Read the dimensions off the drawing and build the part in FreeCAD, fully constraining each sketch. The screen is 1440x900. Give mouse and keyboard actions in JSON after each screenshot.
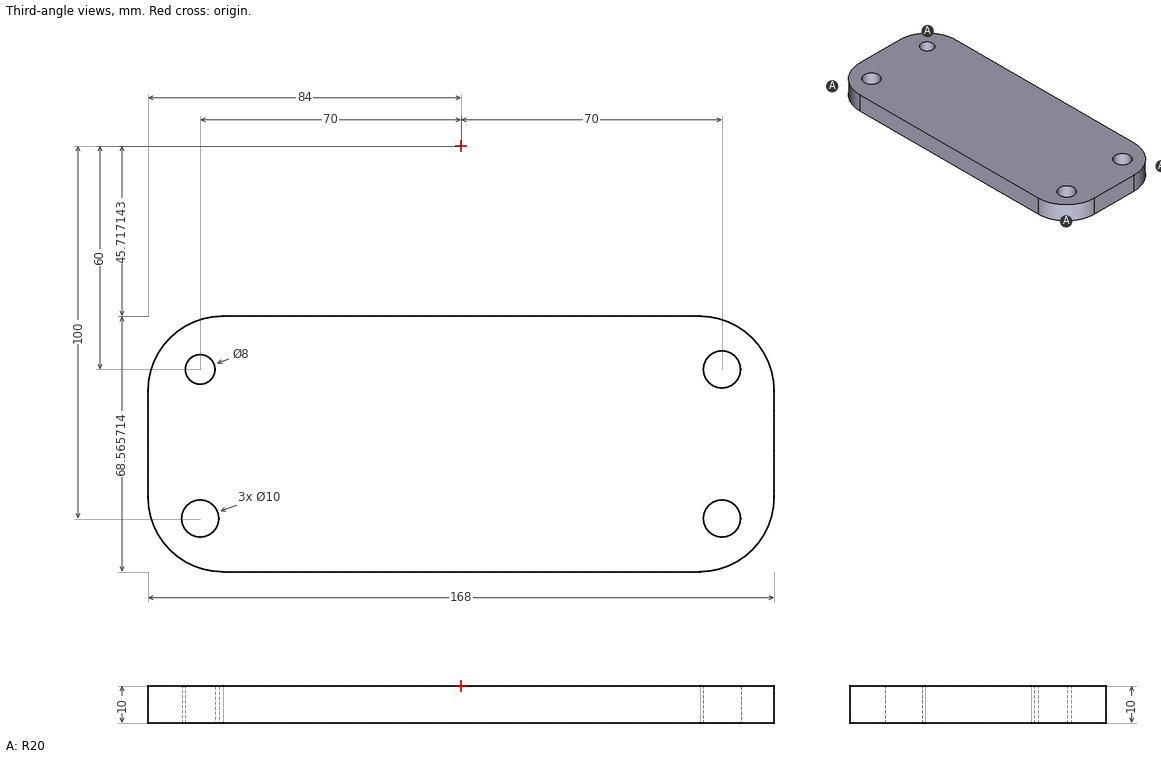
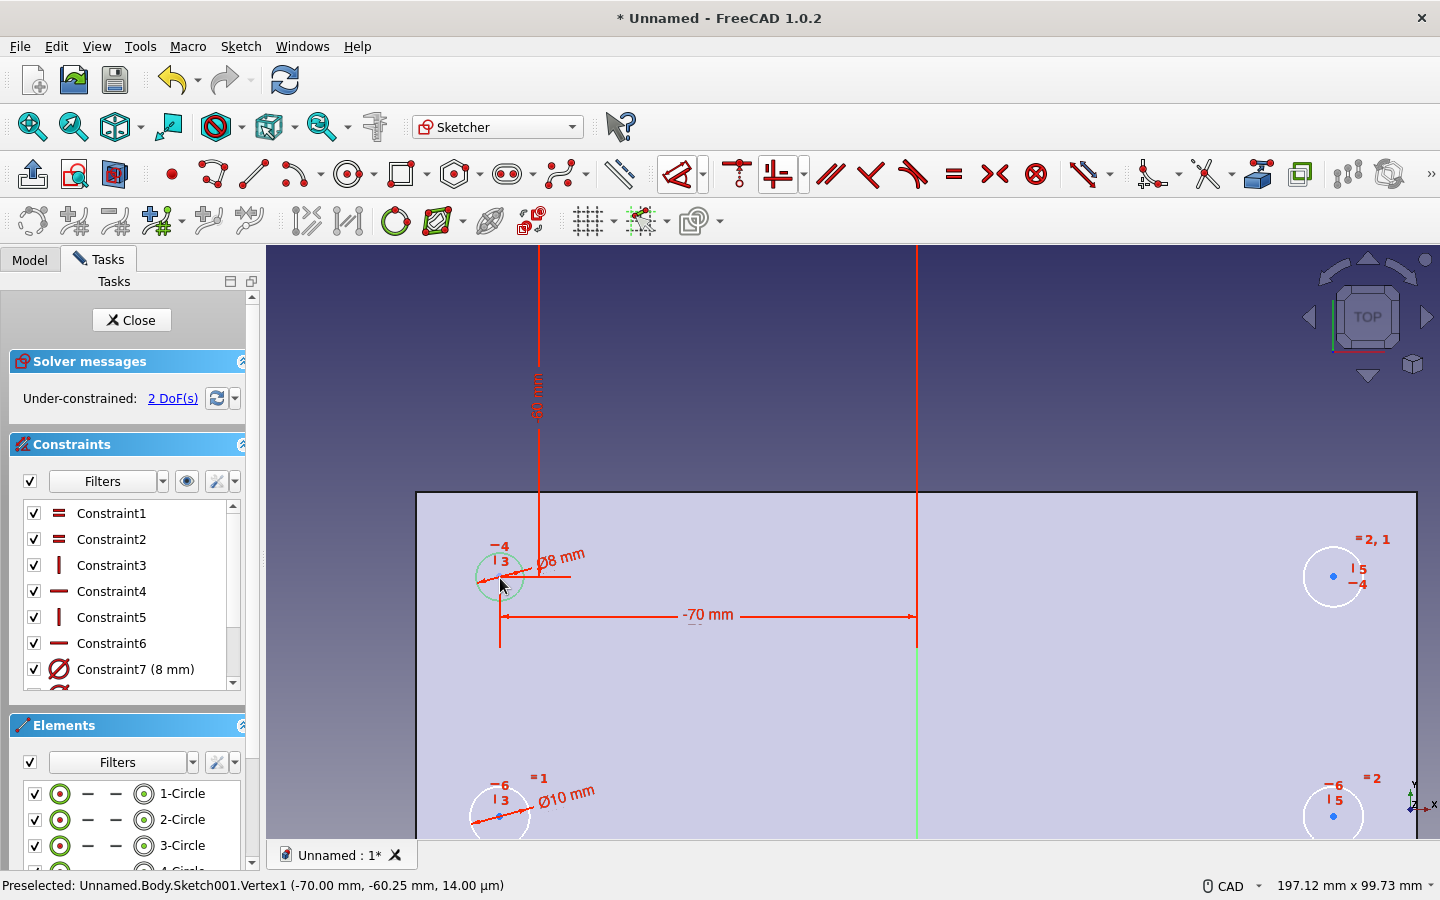
{"action": "scroll", "coordinate": [516, 562], "scroll_direction": "down", "scroll_amount": 2}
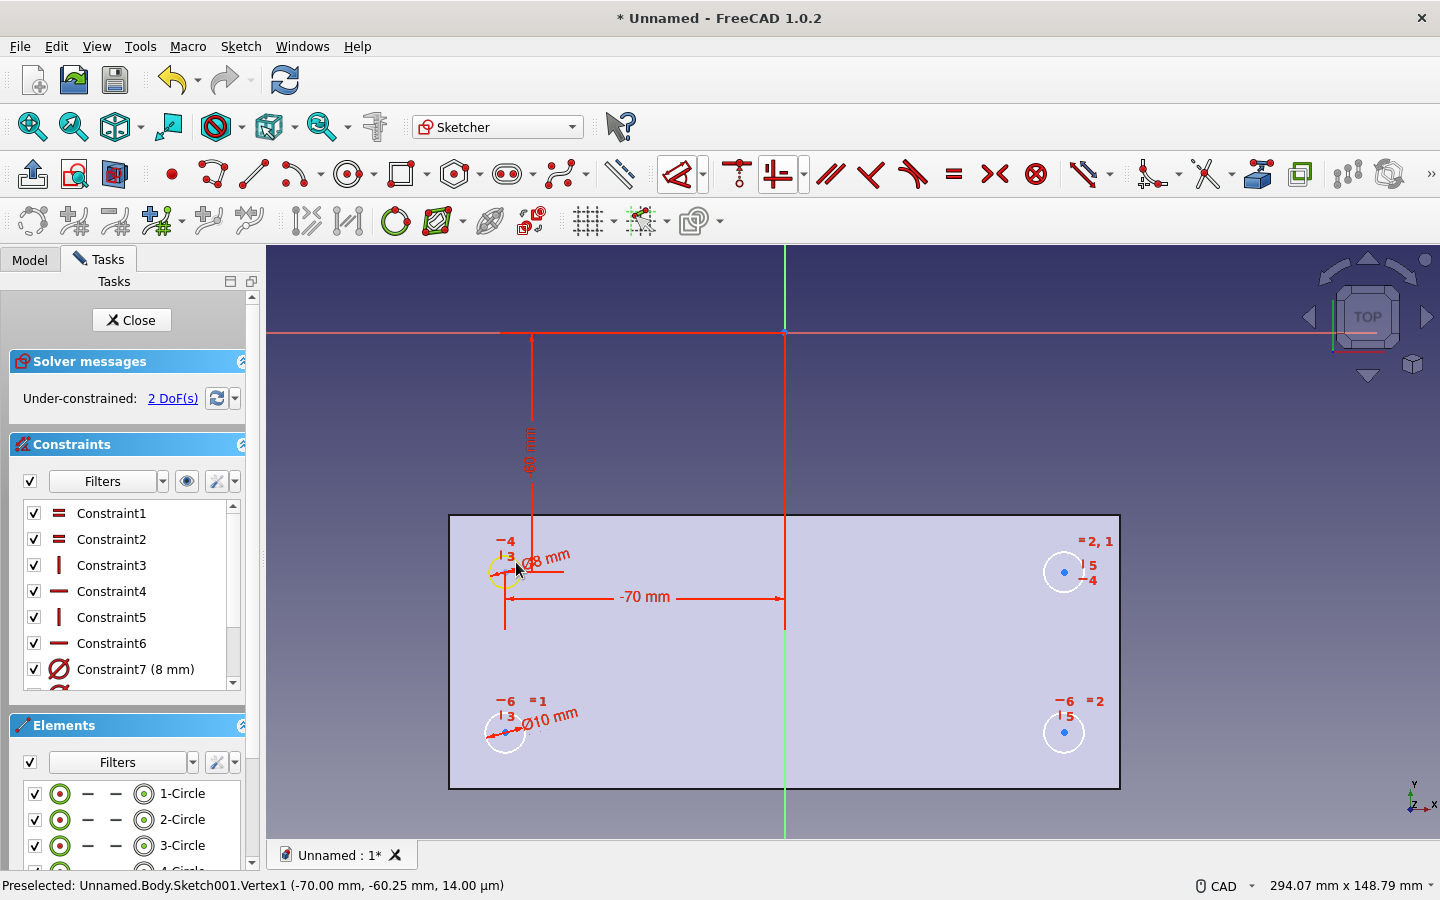
{"action": "left_click", "coordinate": [1064, 572]}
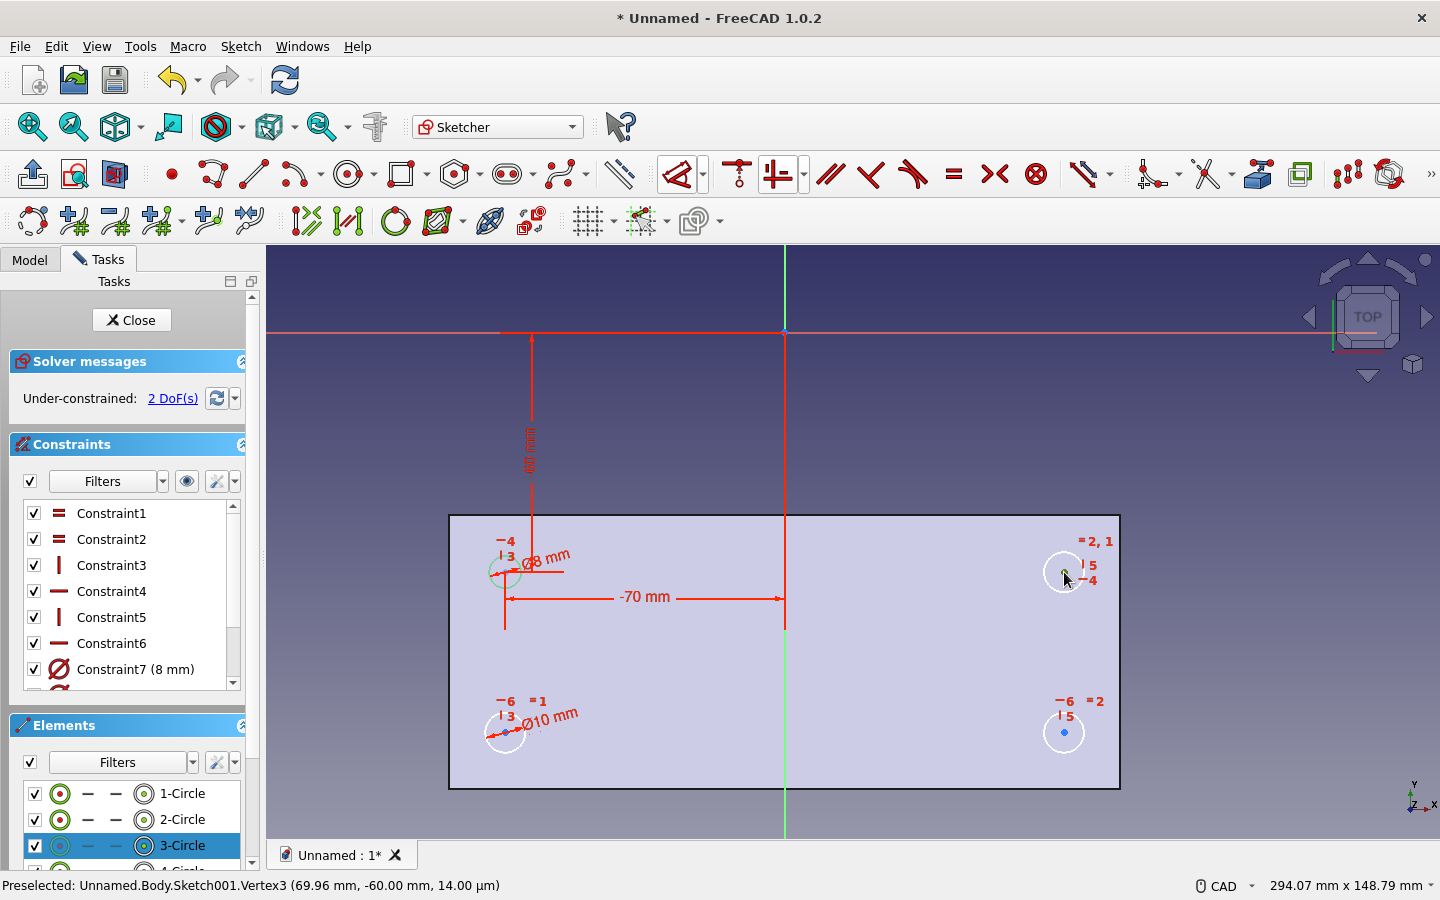
{"action": "left_click", "coordinate": [702, 174]}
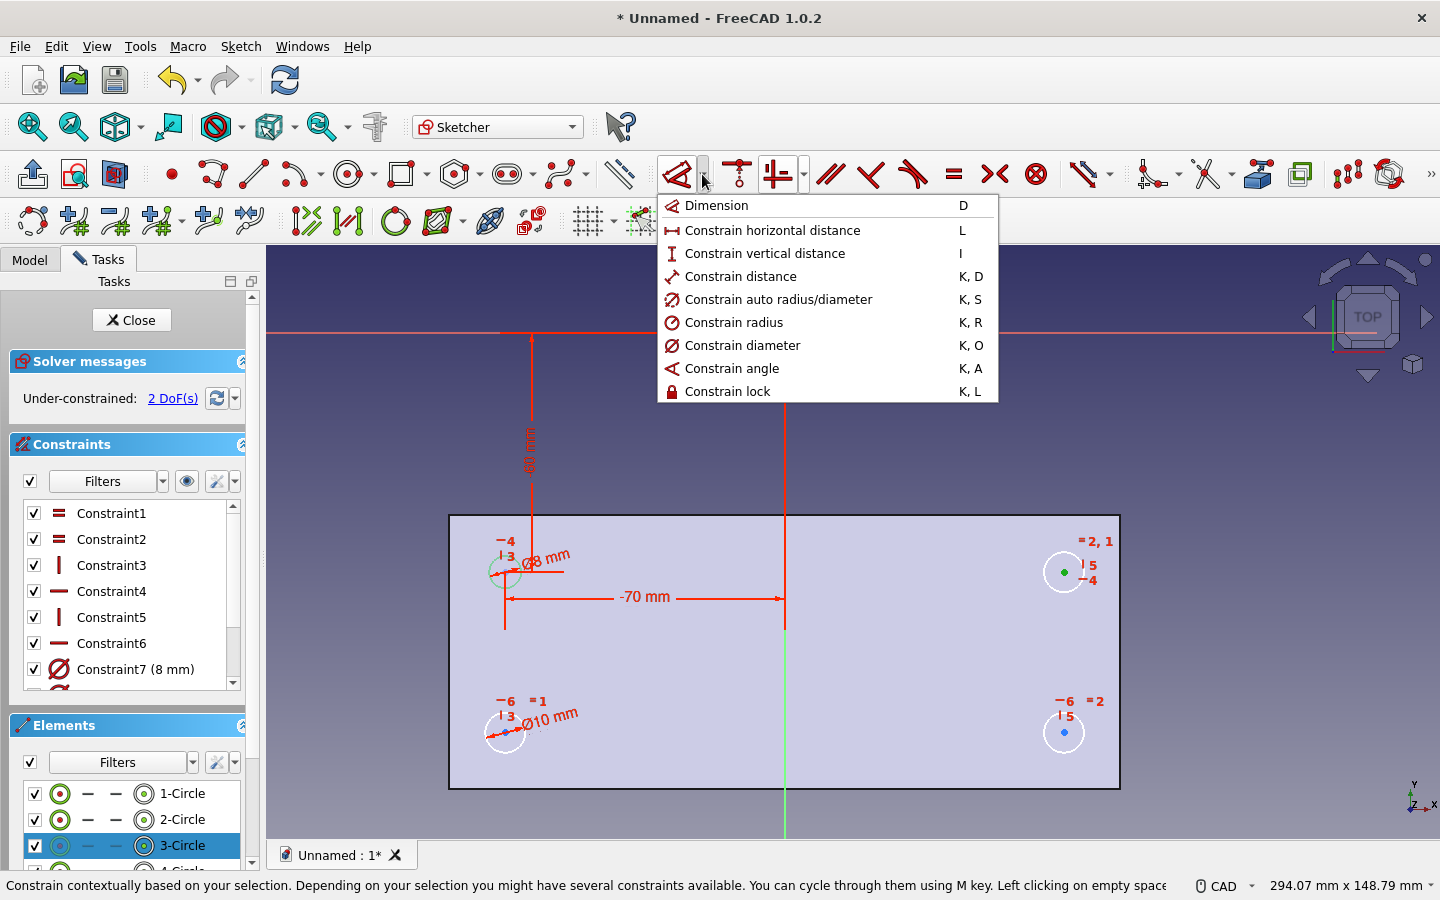
{"action": "left_click", "coordinate": [828, 230]}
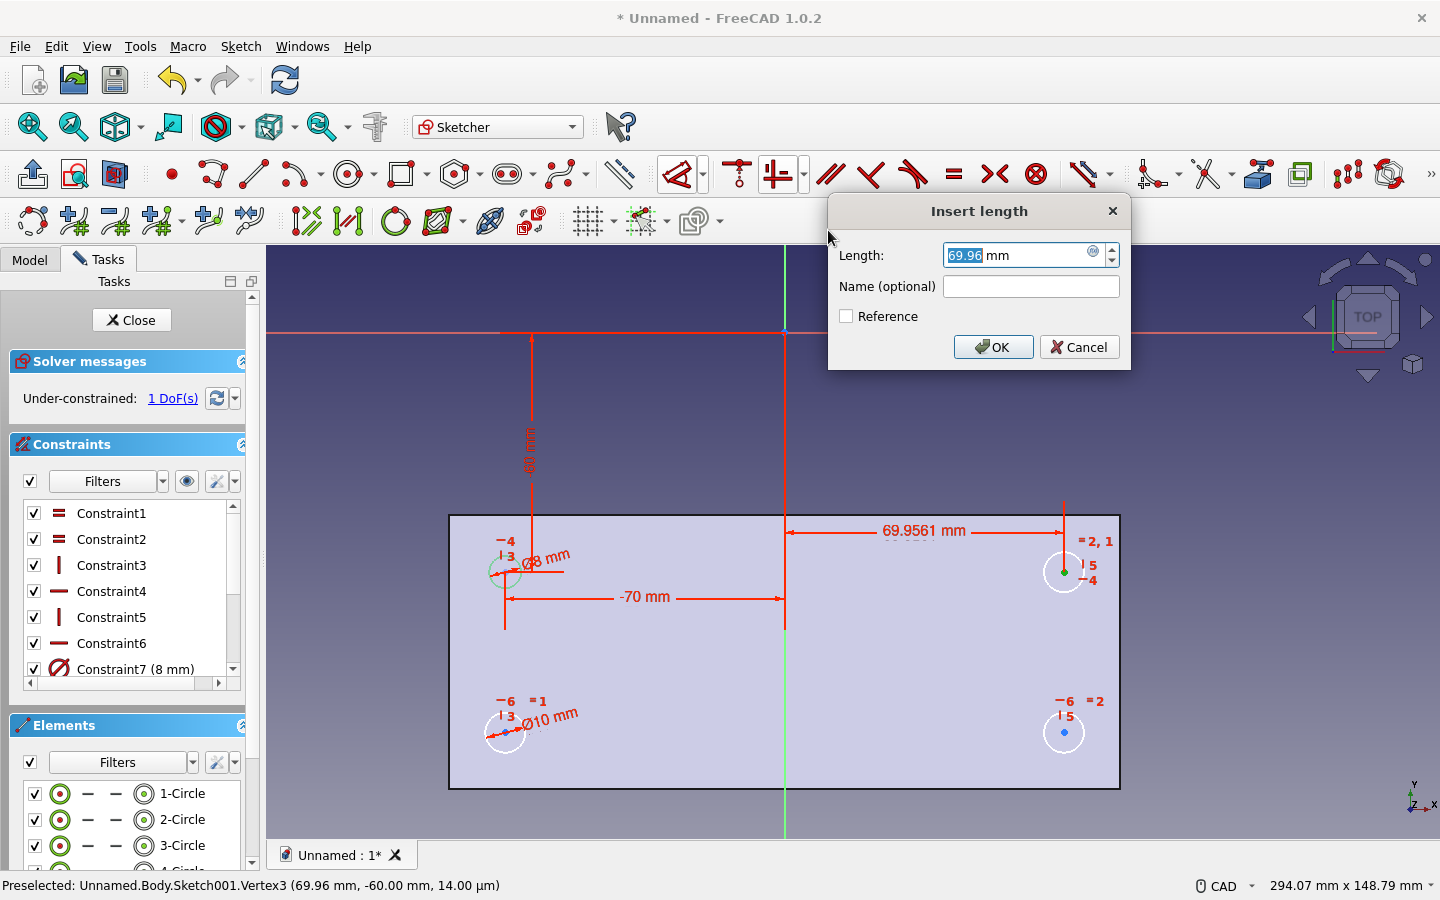
{"action": "type", "text": "70"}
{"action": "key", "text": "Return"}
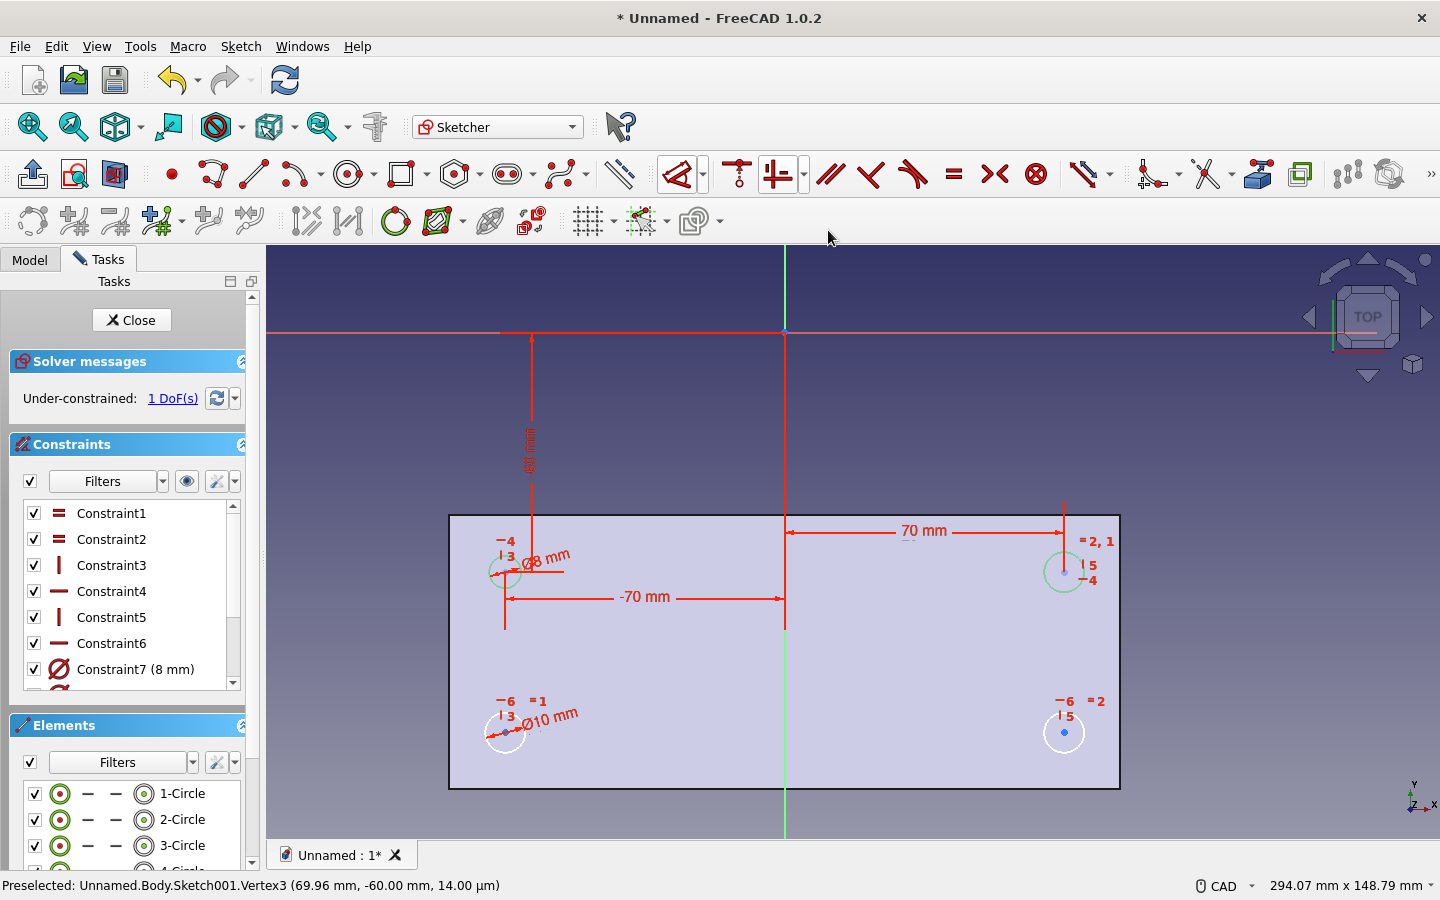
{"action": "left_click", "coordinate": [505, 733]}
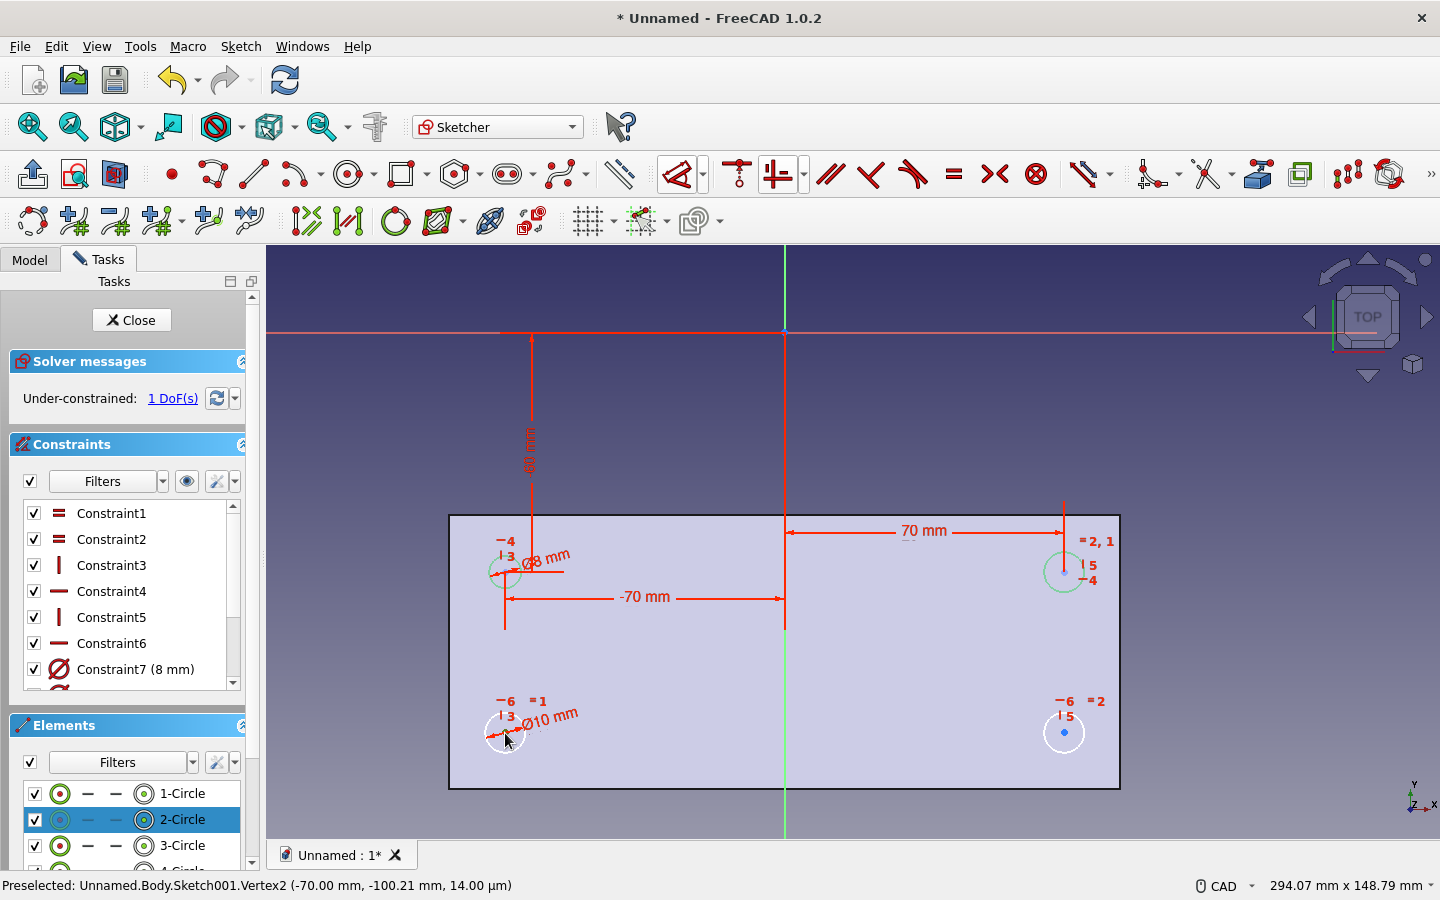
{"action": "key", "text": "i"}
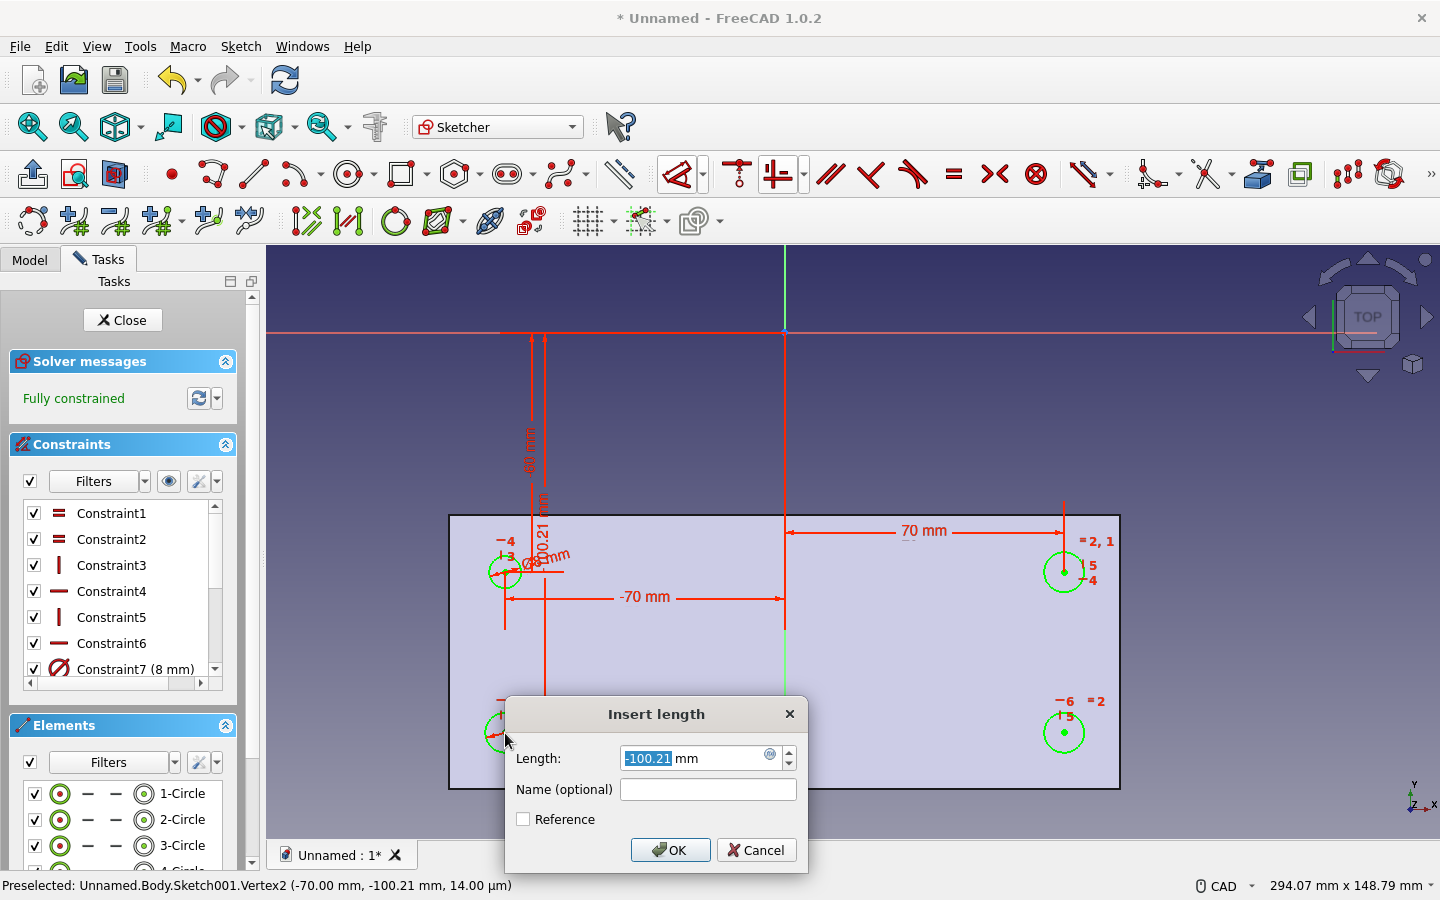
{"action": "type", "text": "-100"}
{"action": "key", "text": "Return"}